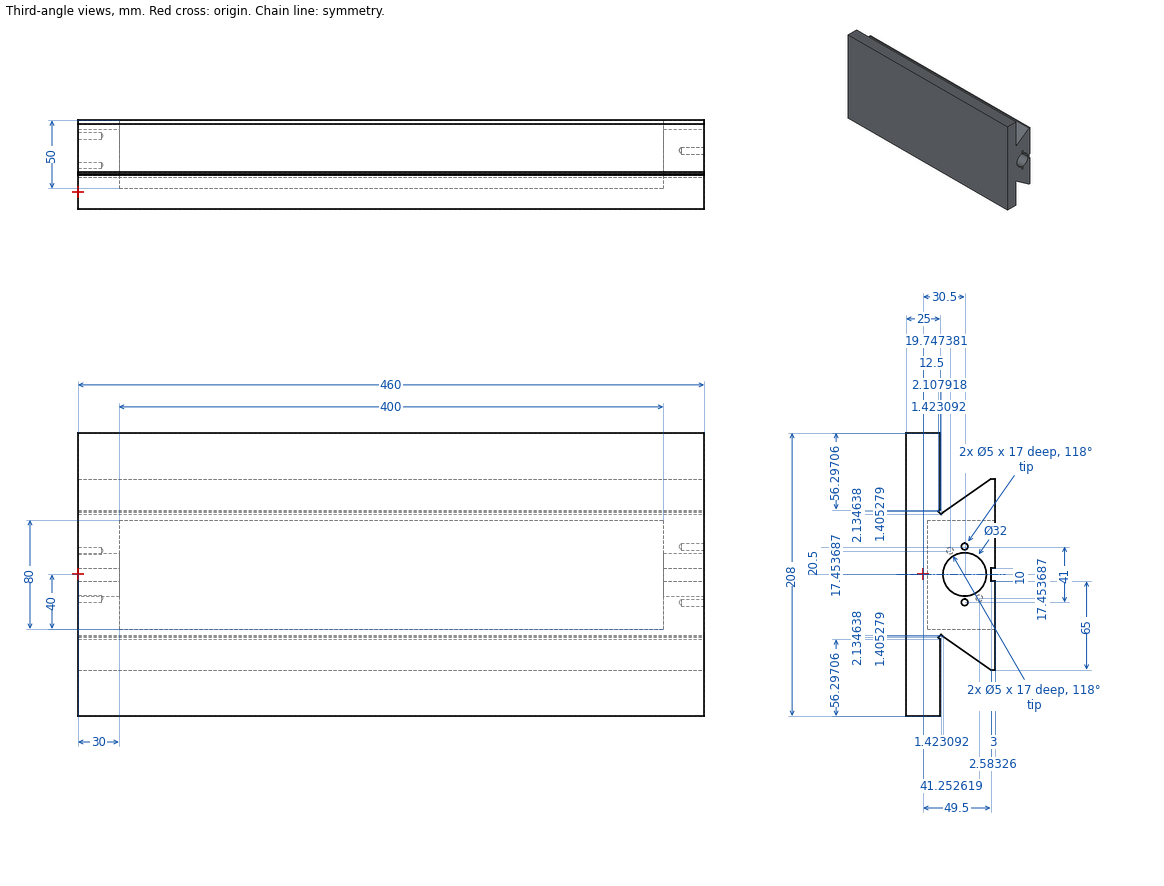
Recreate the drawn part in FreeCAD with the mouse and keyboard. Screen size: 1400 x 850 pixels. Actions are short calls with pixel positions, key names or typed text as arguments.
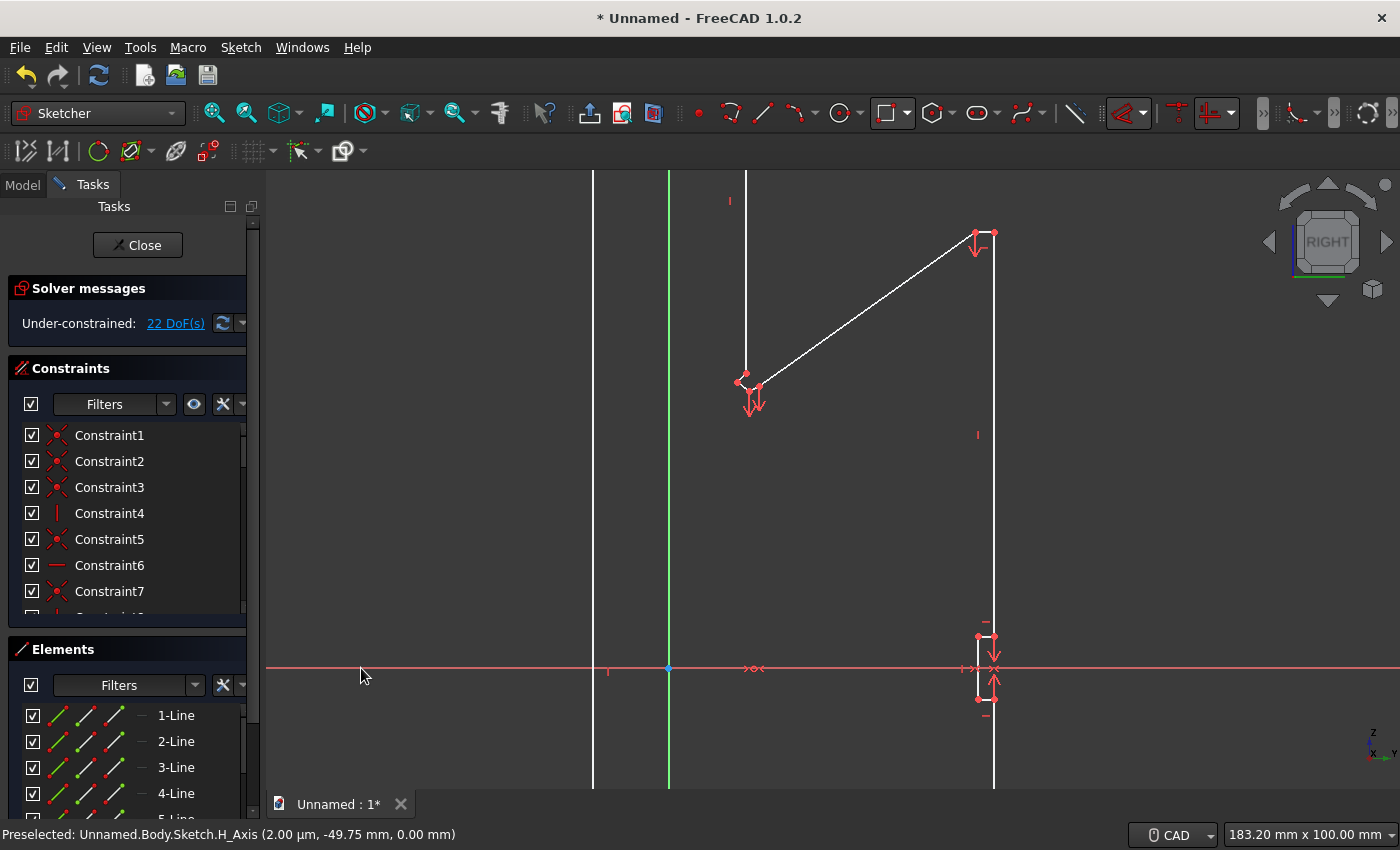
scroll(752, 398, down, 6)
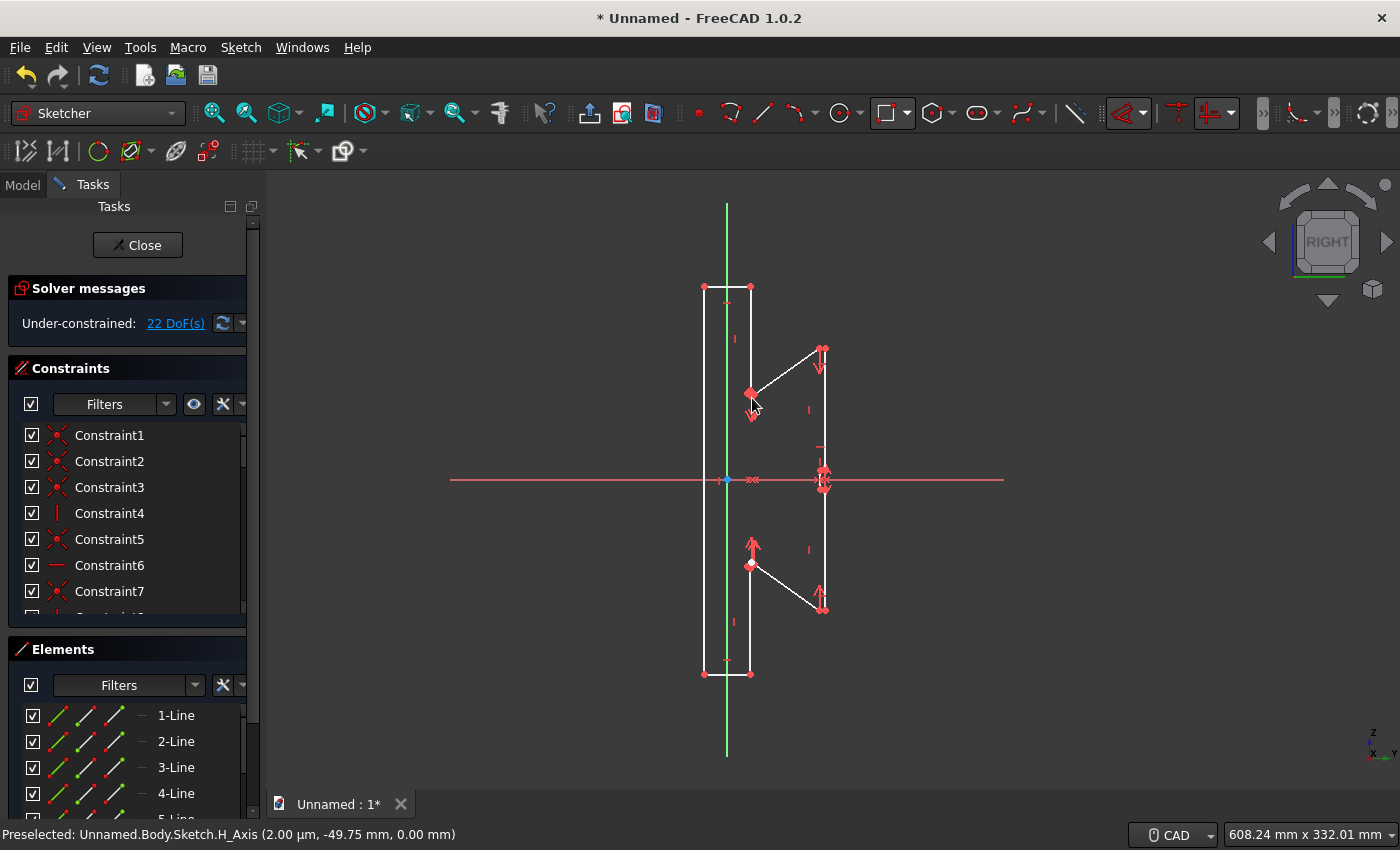
click(751, 287)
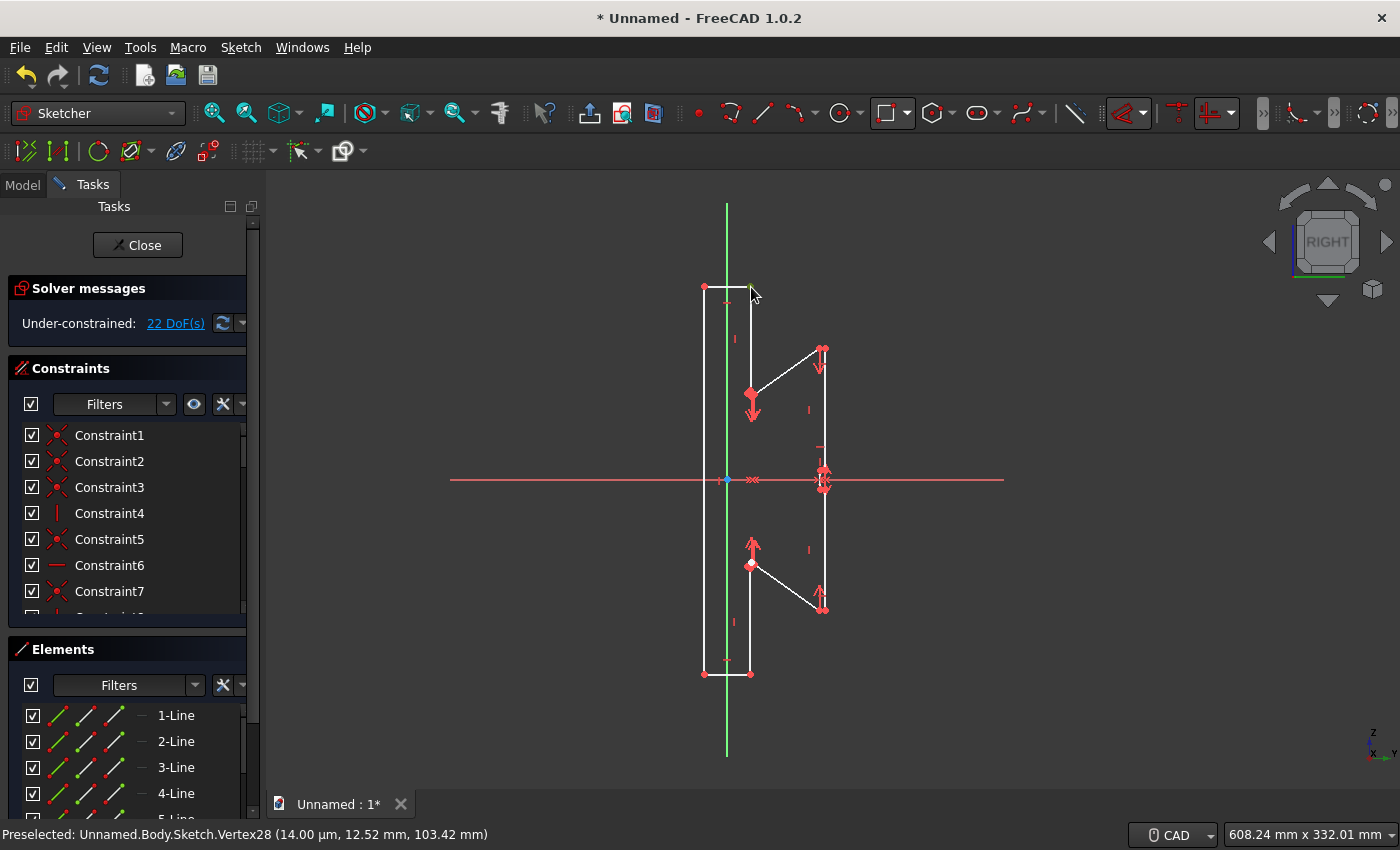
click(750, 675)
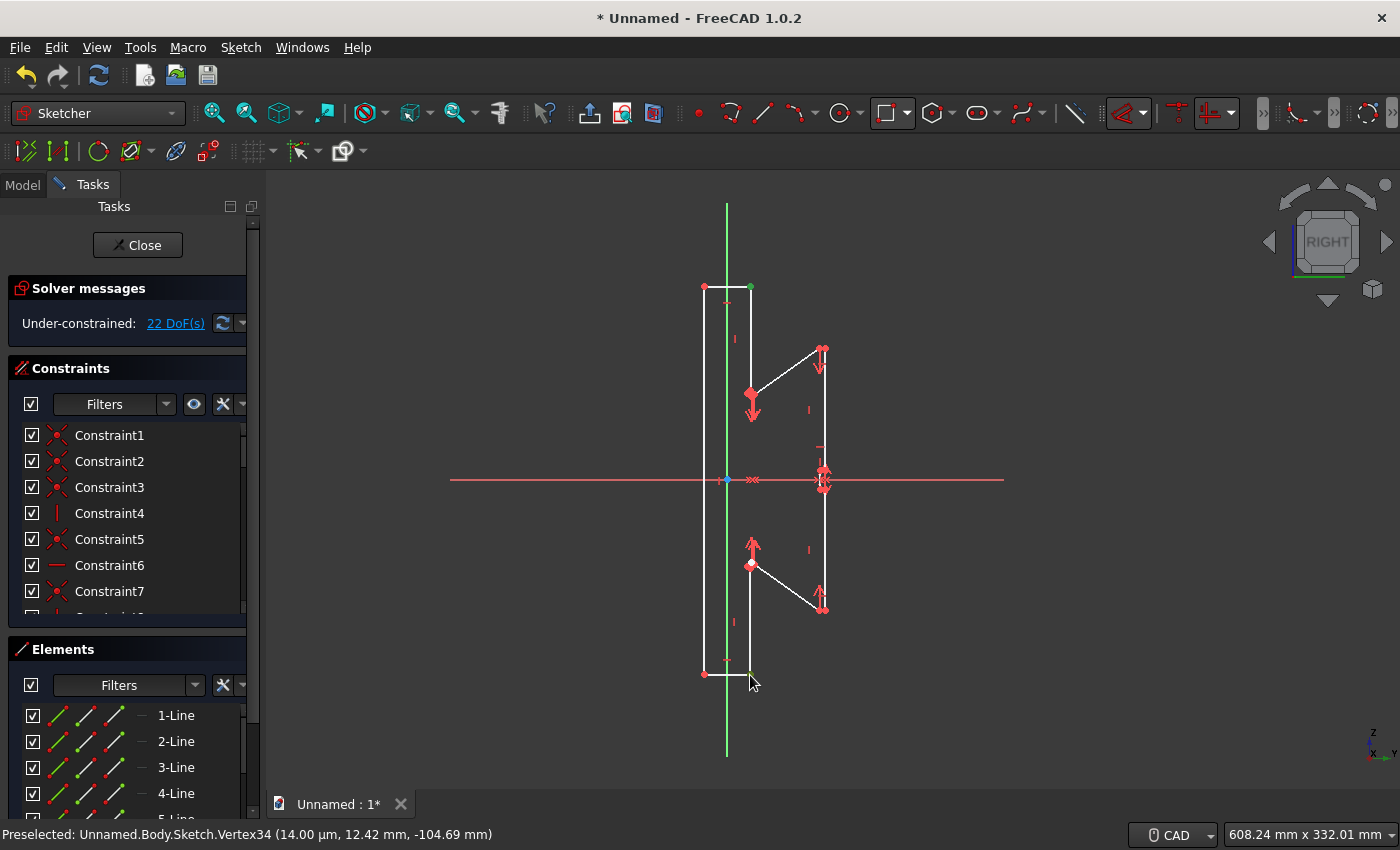
click(496, 480)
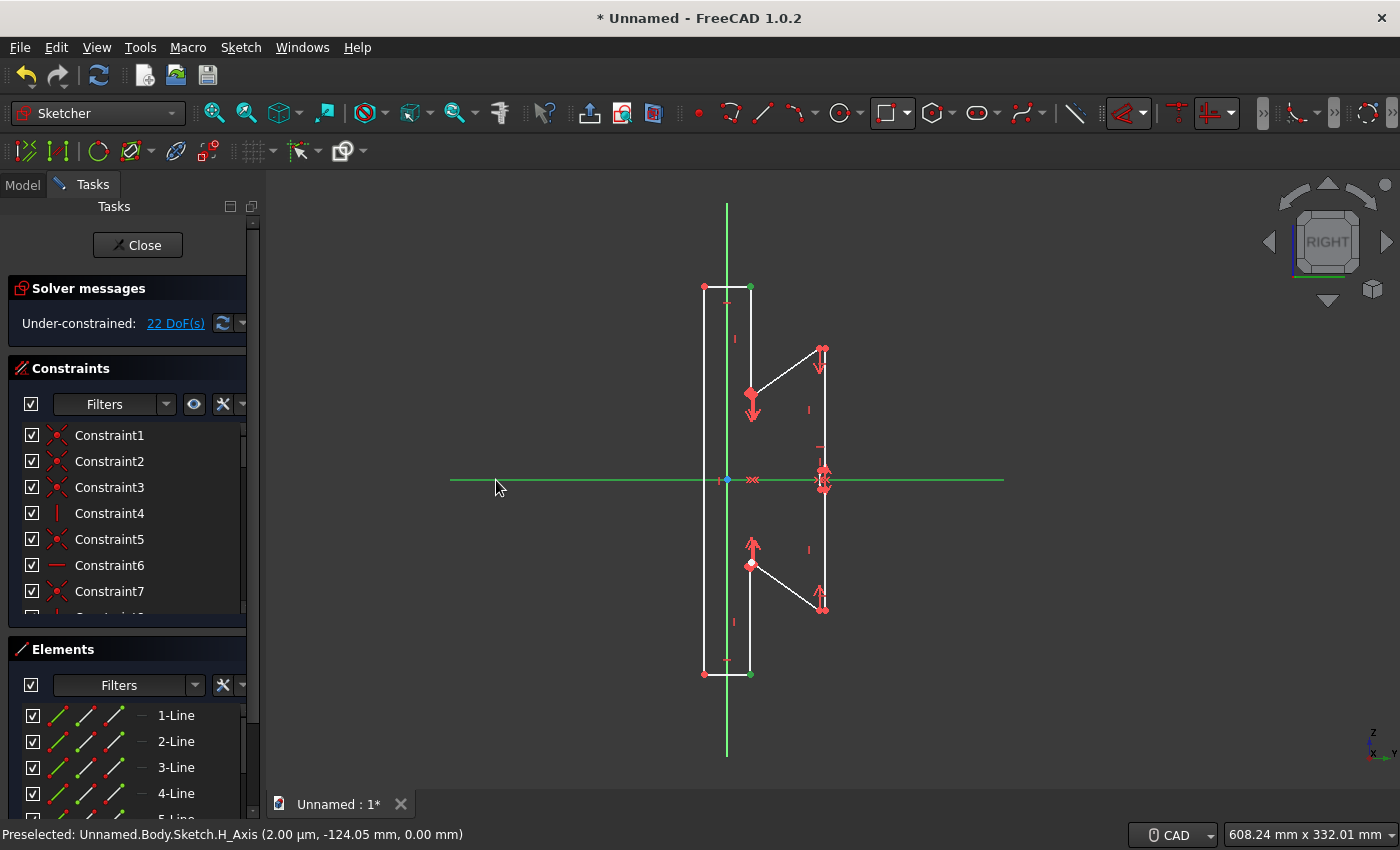
key(s)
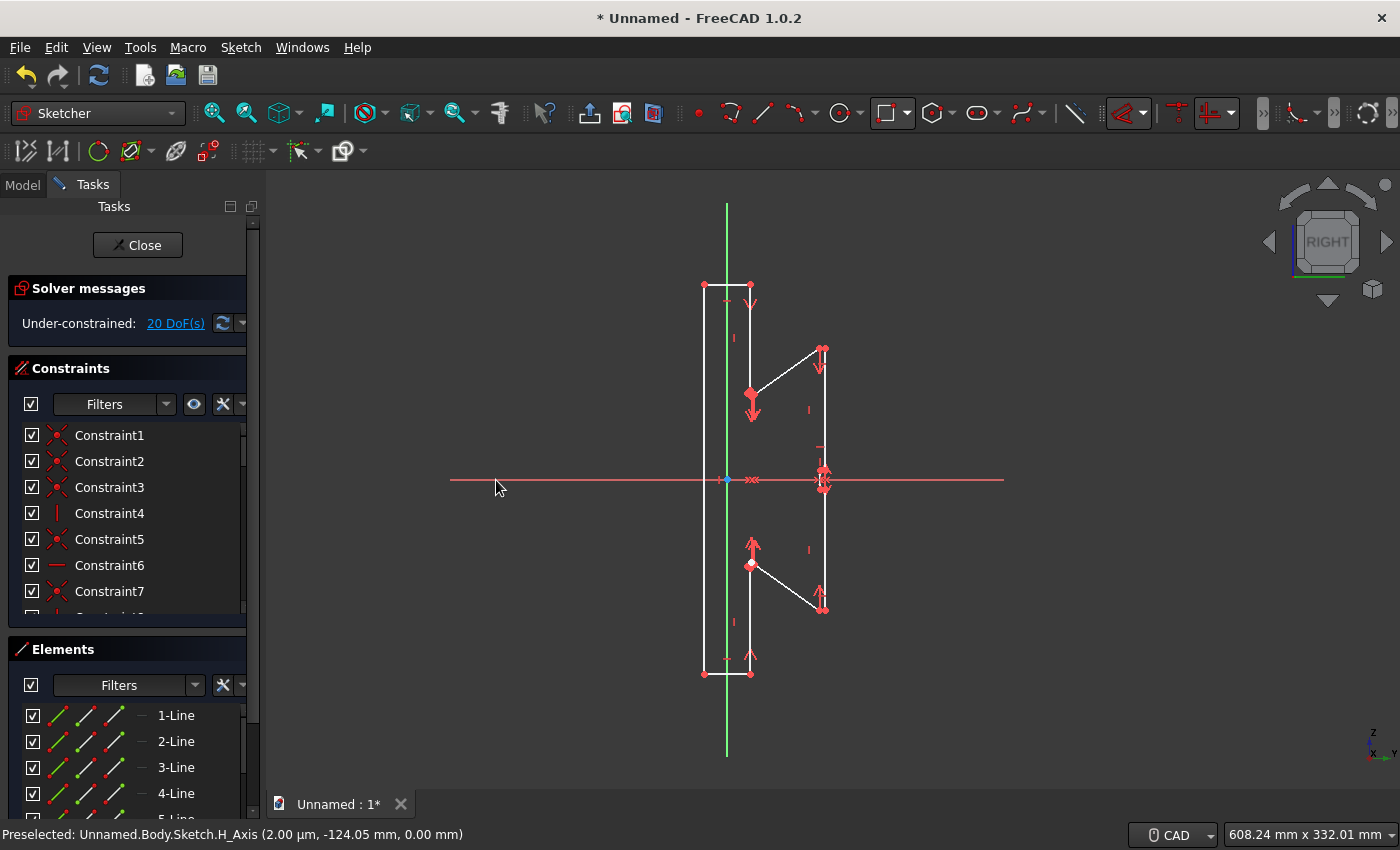
scroll(748, 393, up, 7)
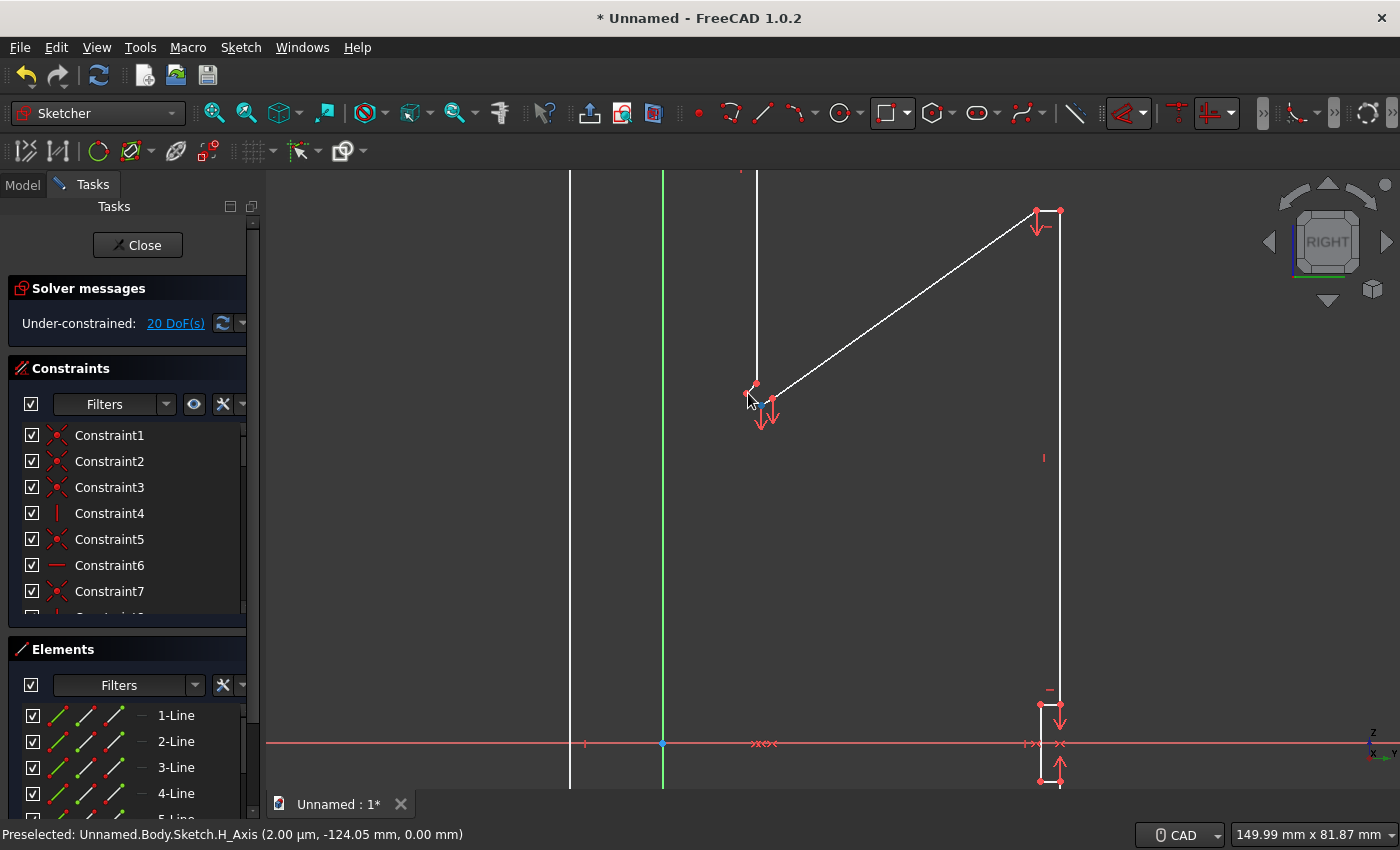
click(747, 394)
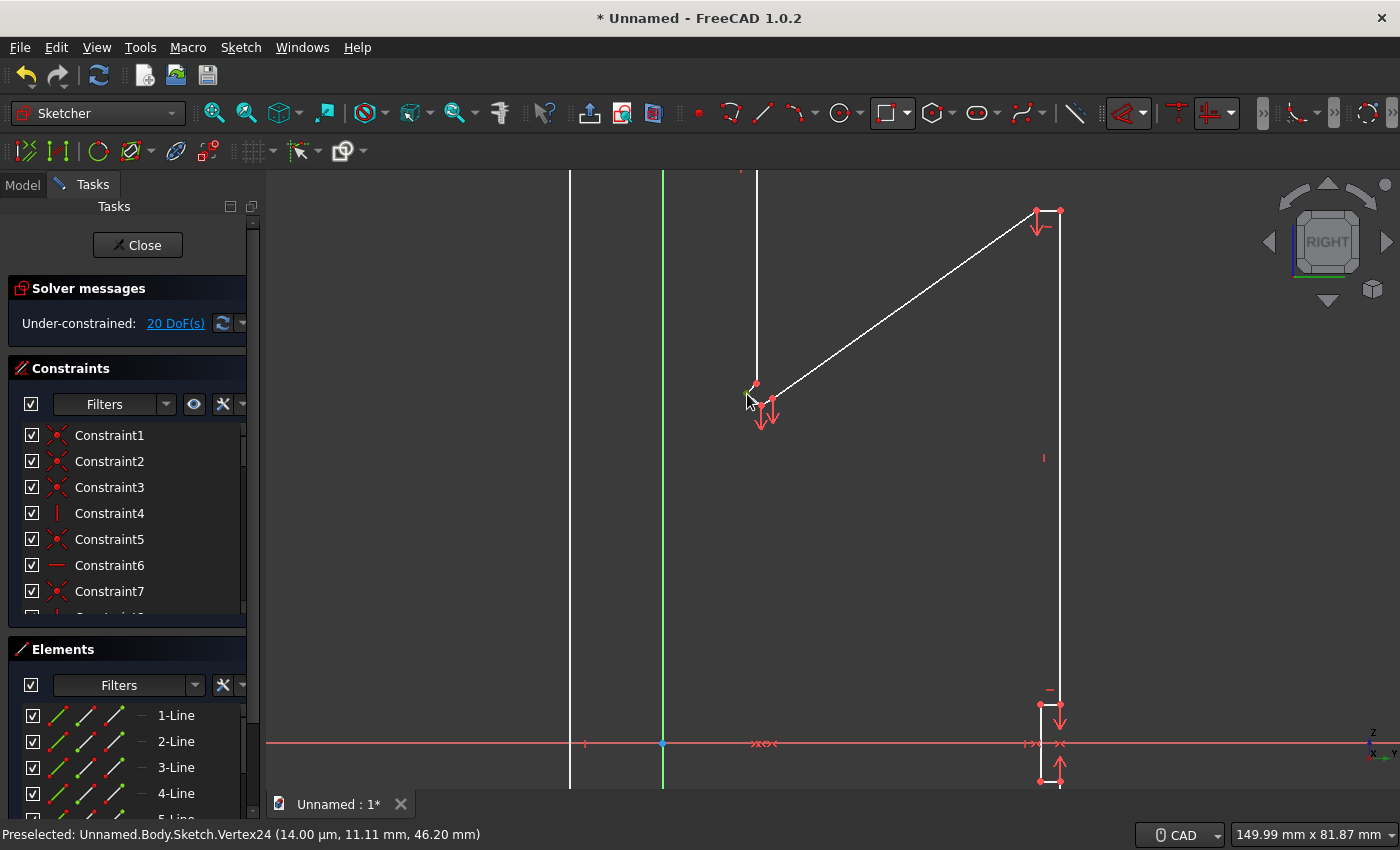
scroll(748, 393, down, 7)